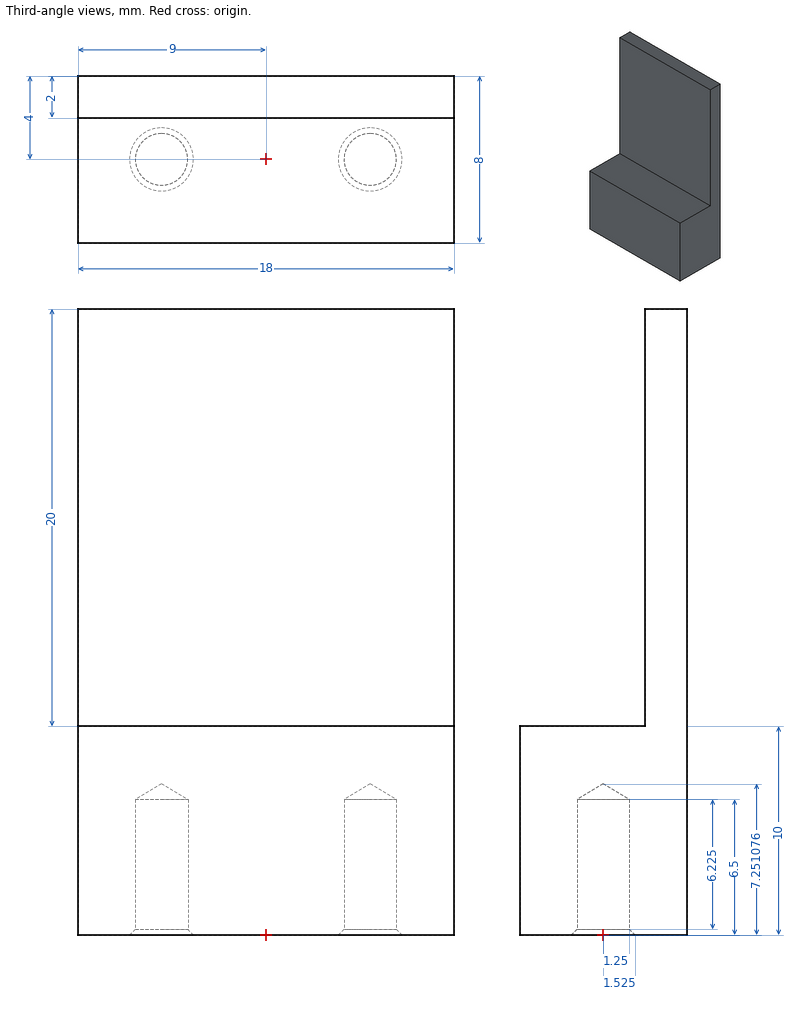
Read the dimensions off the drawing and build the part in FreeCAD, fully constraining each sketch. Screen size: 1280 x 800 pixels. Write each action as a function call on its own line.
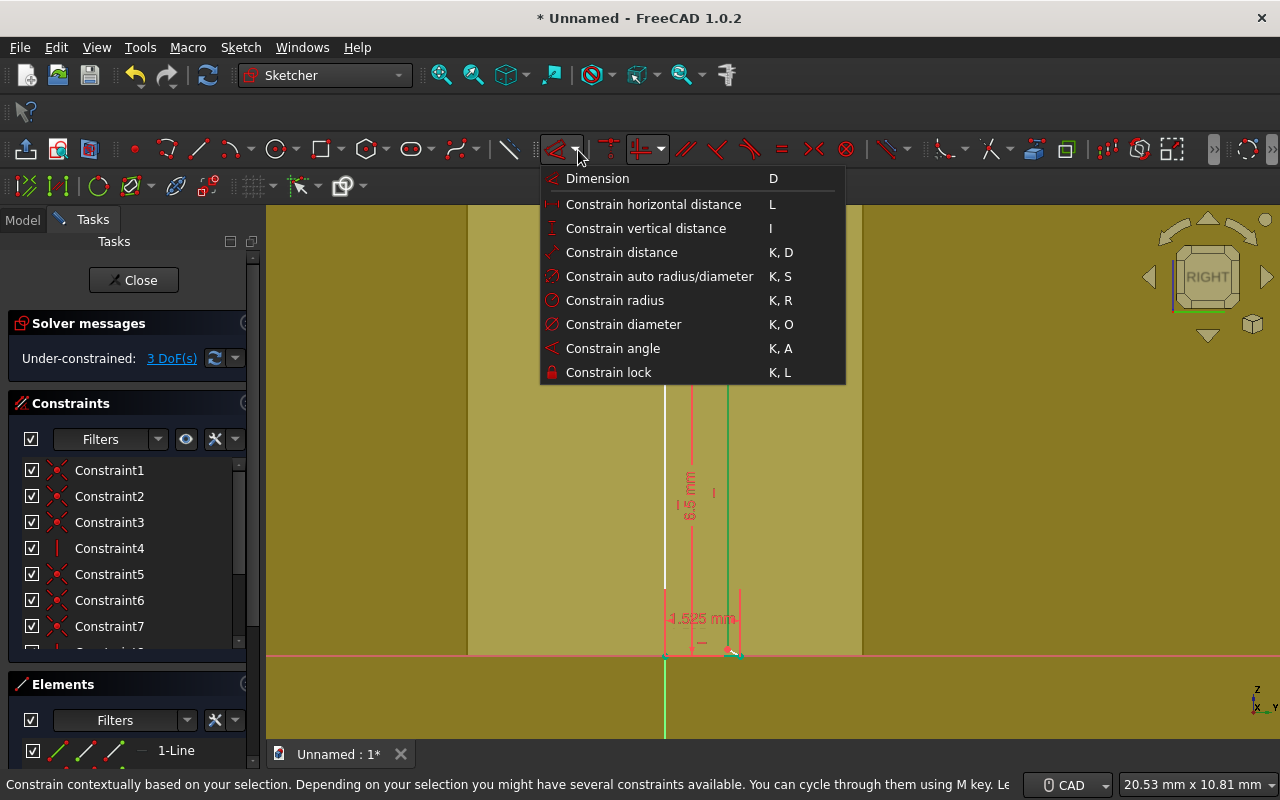
click(693, 228)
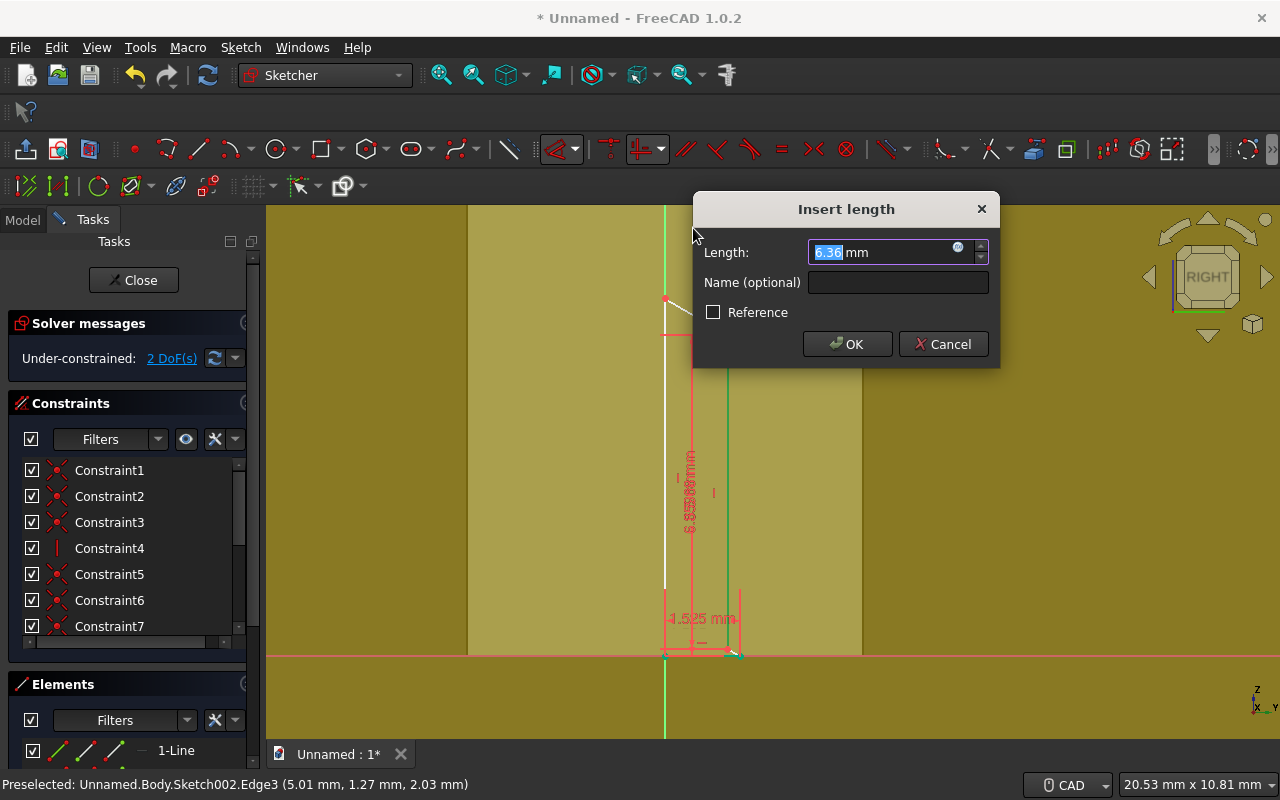
text(6.225)
key(Return)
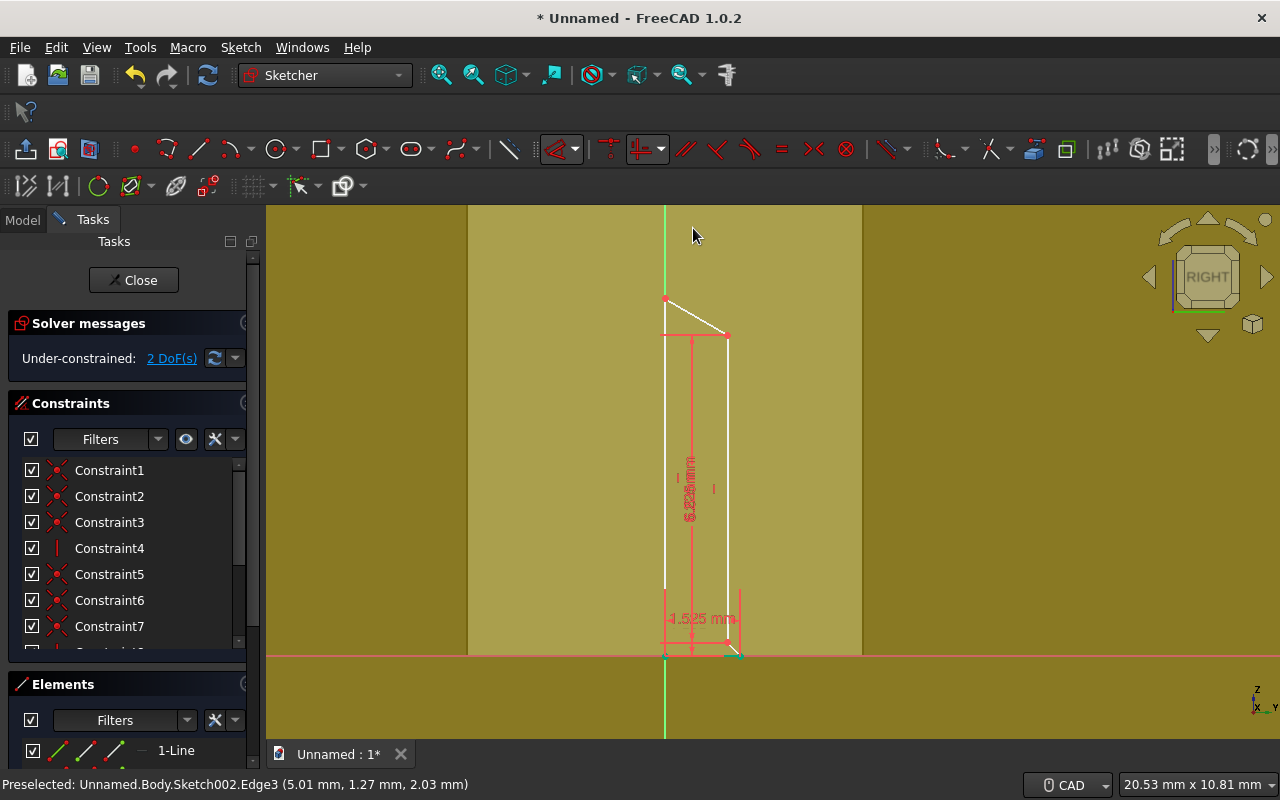
click(728, 643)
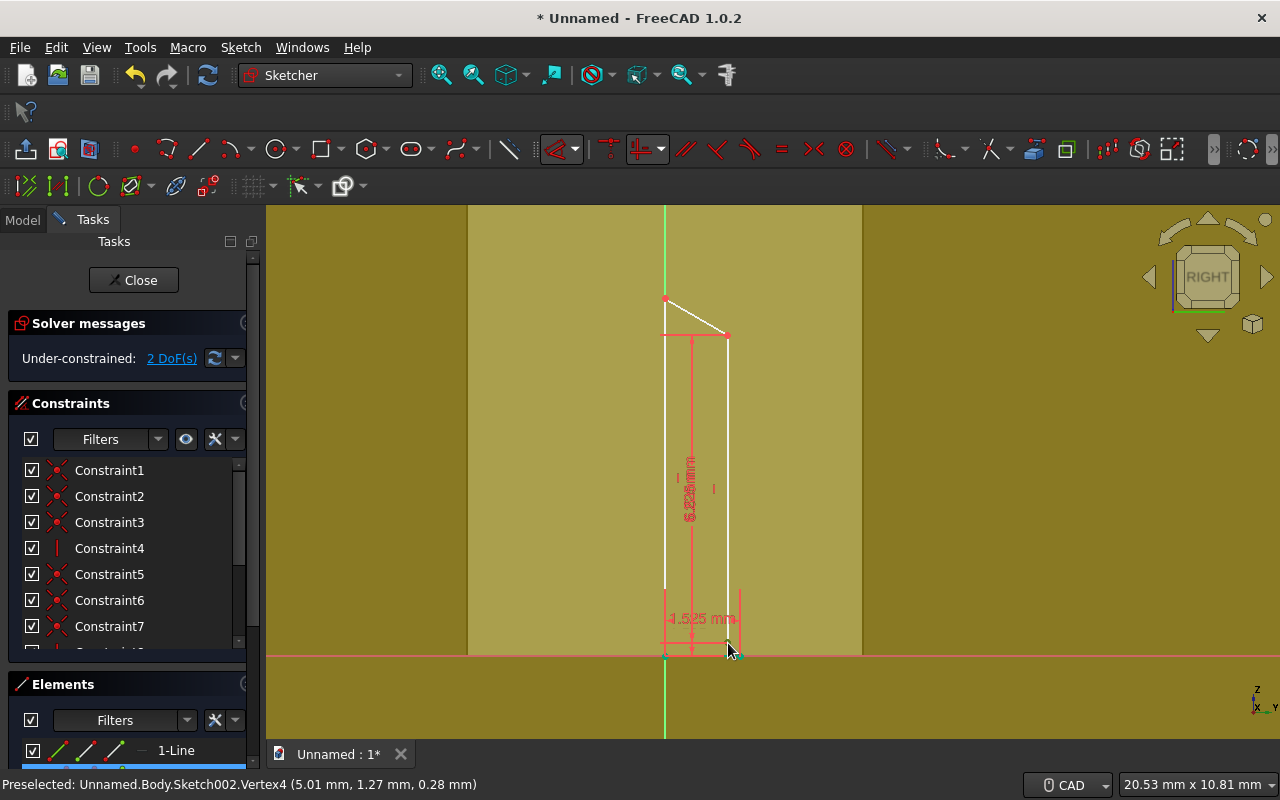
key(l)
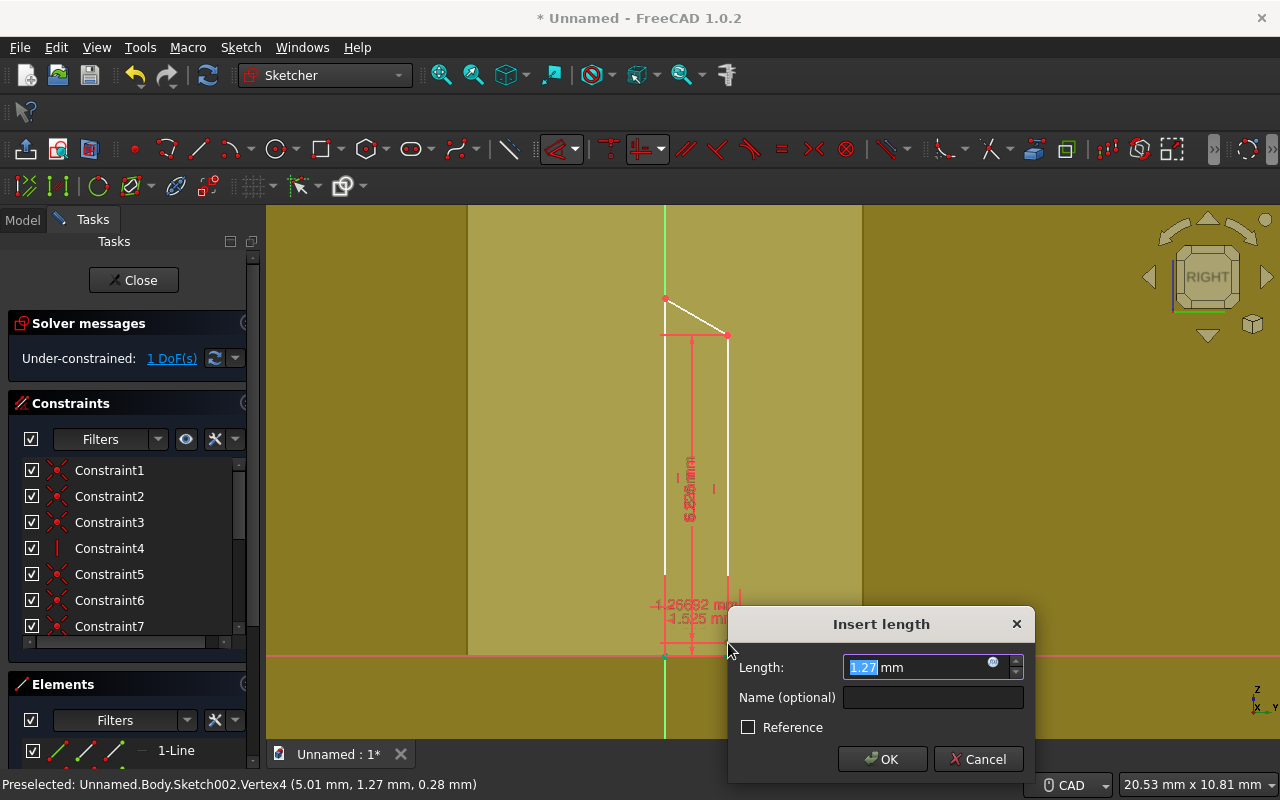
text(1.25)
key(Return)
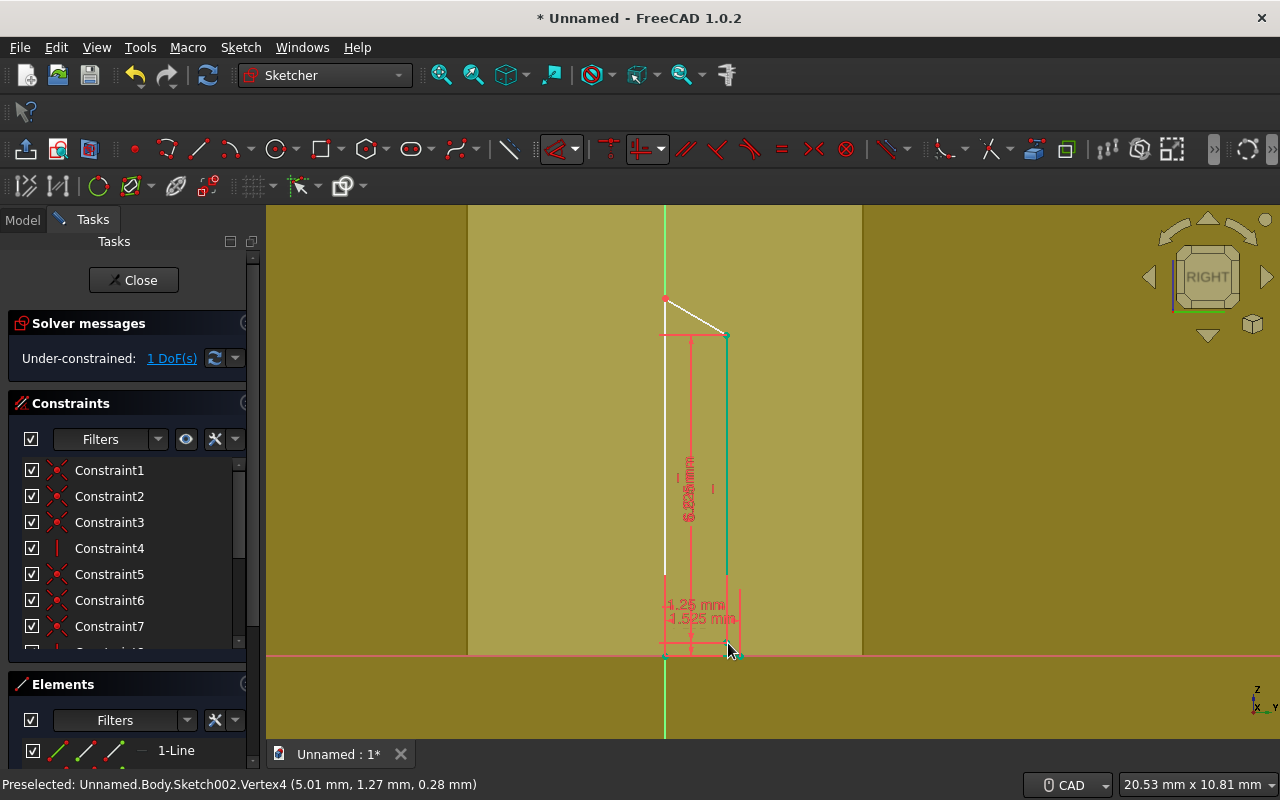
click(665, 406)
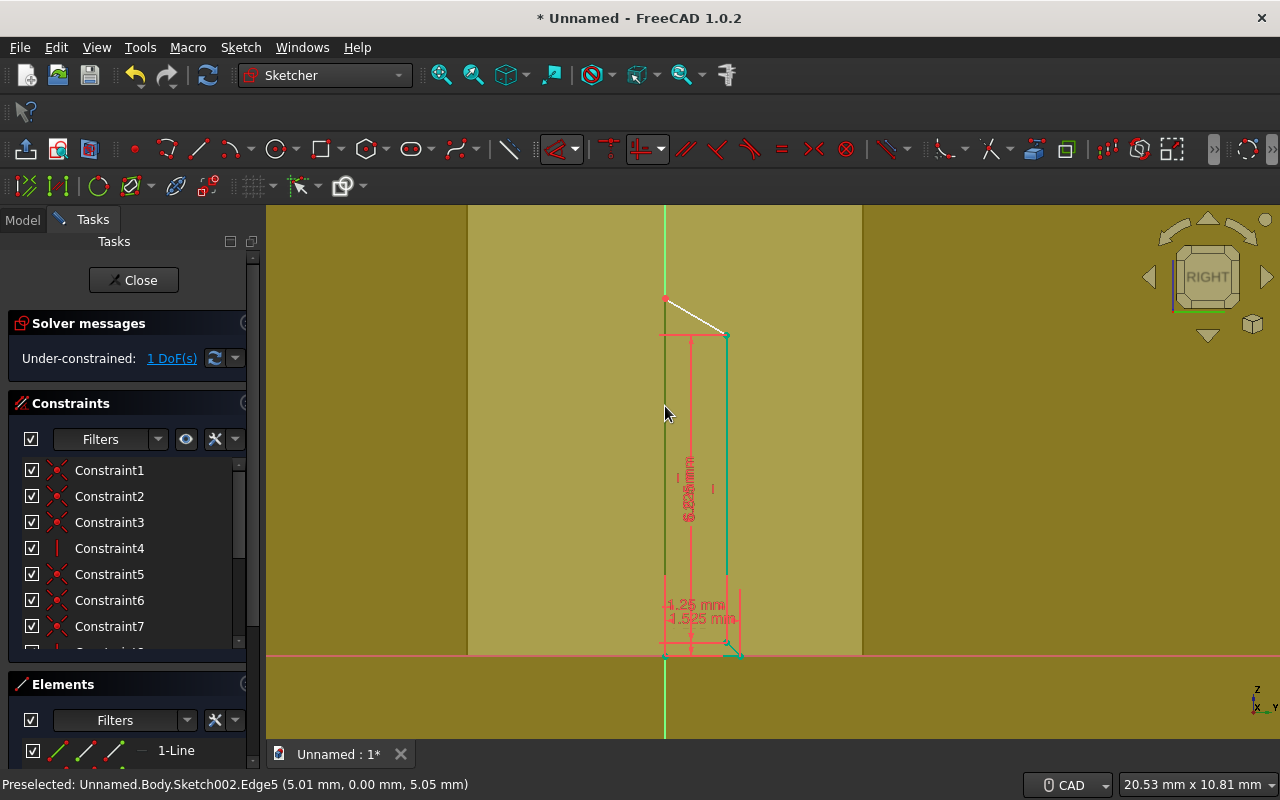
click(578, 150)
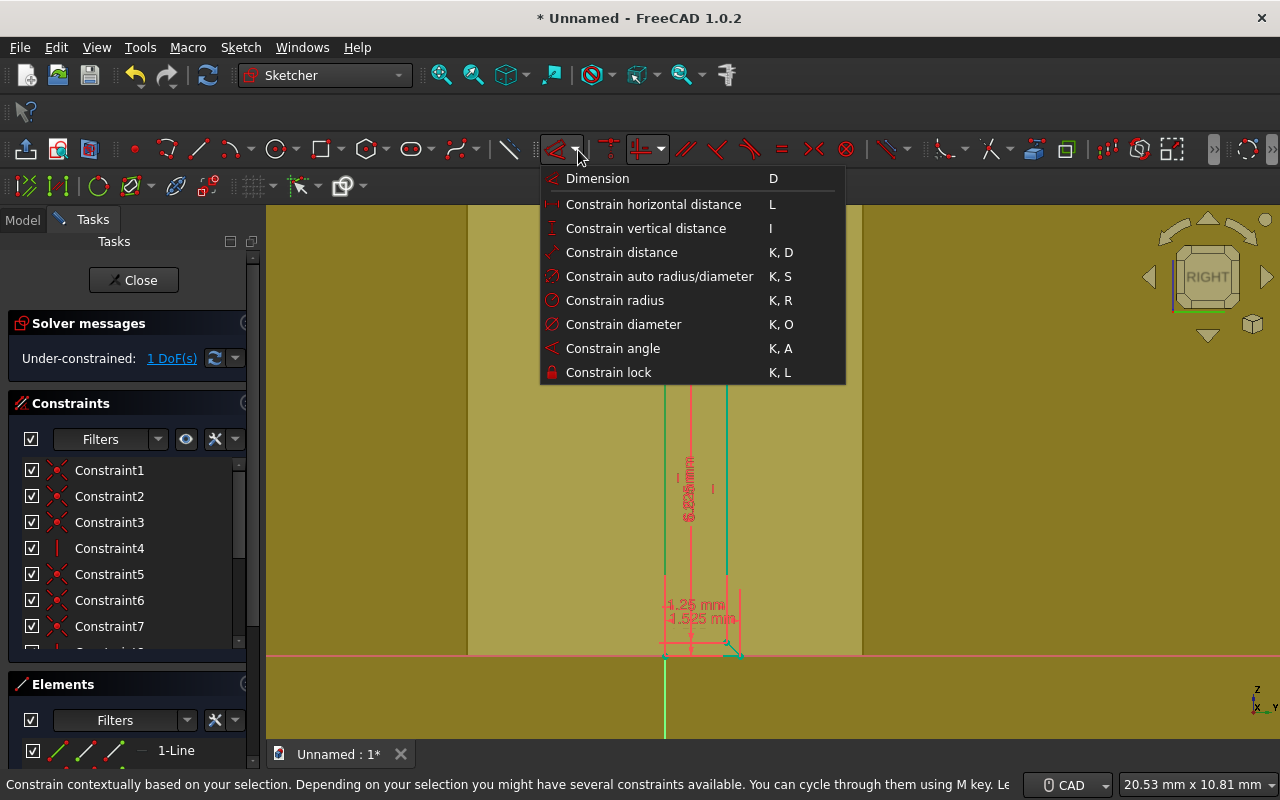
click(693, 228)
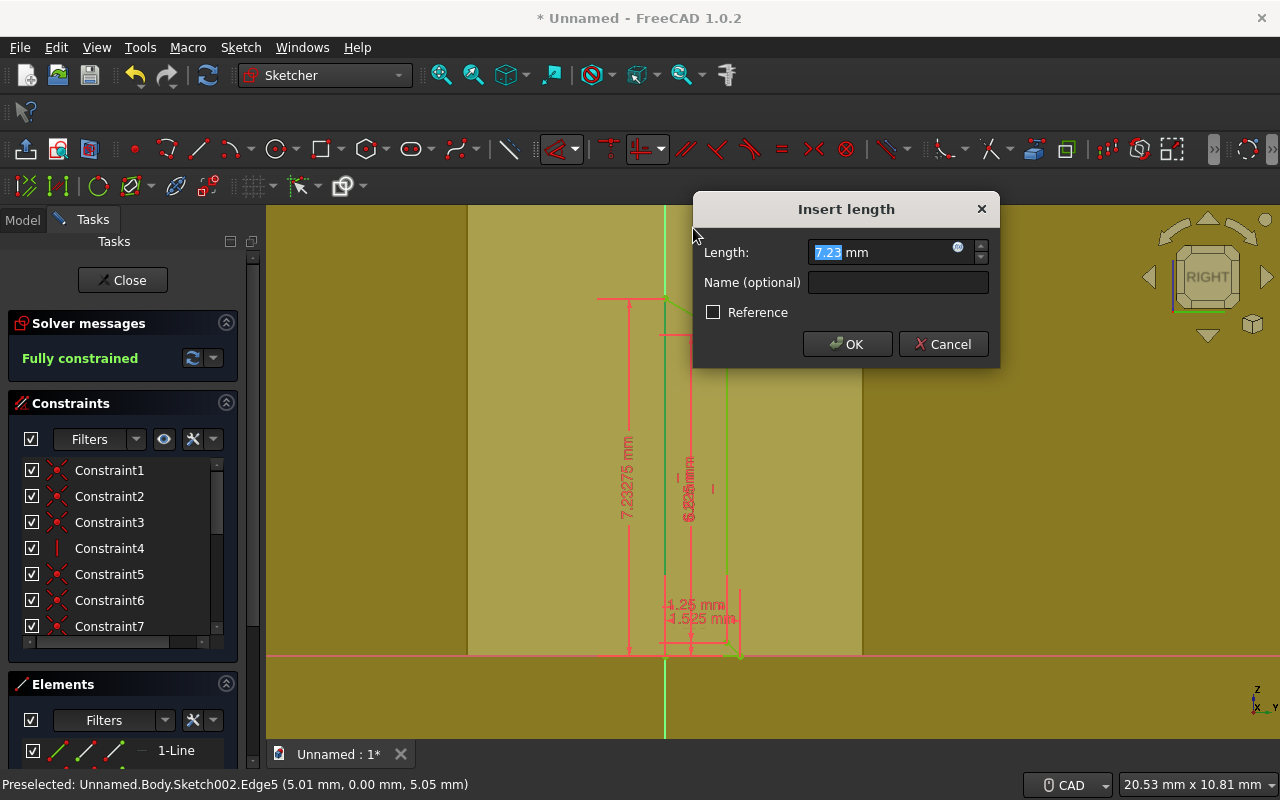
text(7.251076)
key(Return)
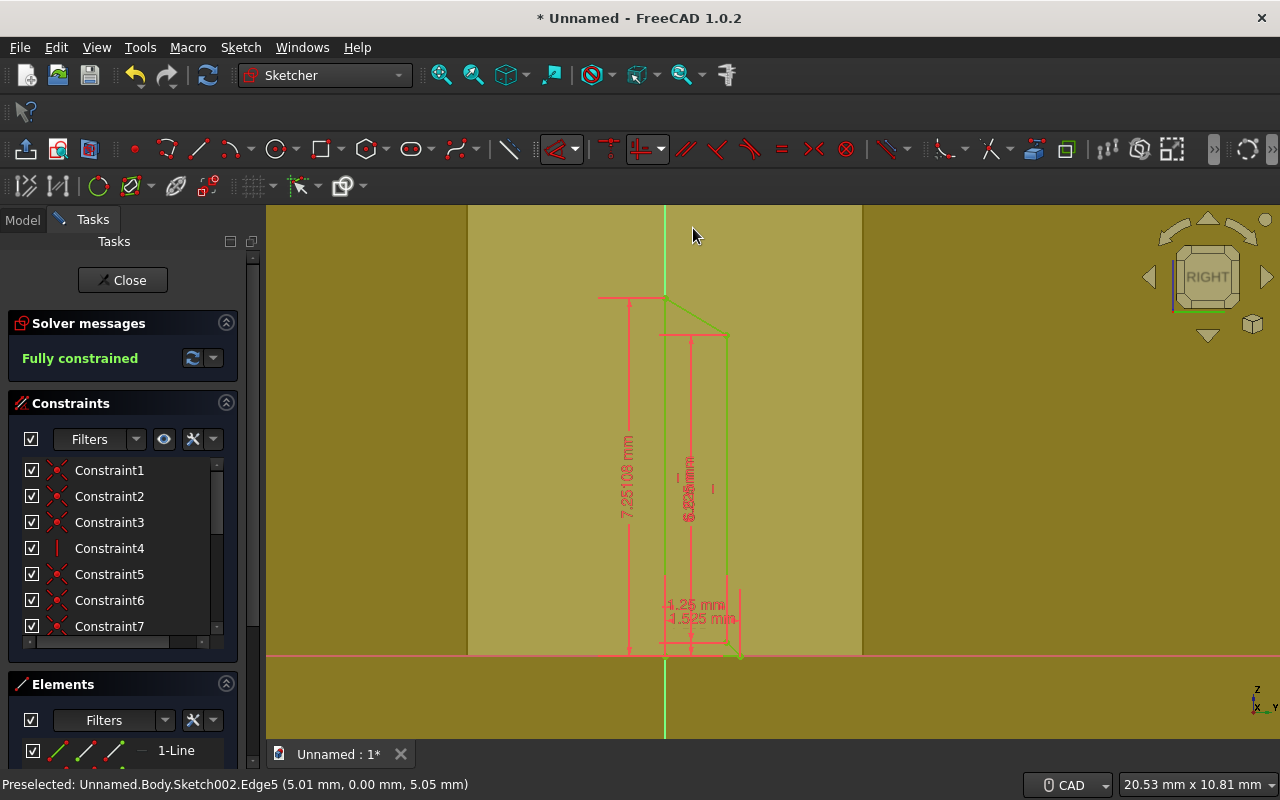
click(123, 280)